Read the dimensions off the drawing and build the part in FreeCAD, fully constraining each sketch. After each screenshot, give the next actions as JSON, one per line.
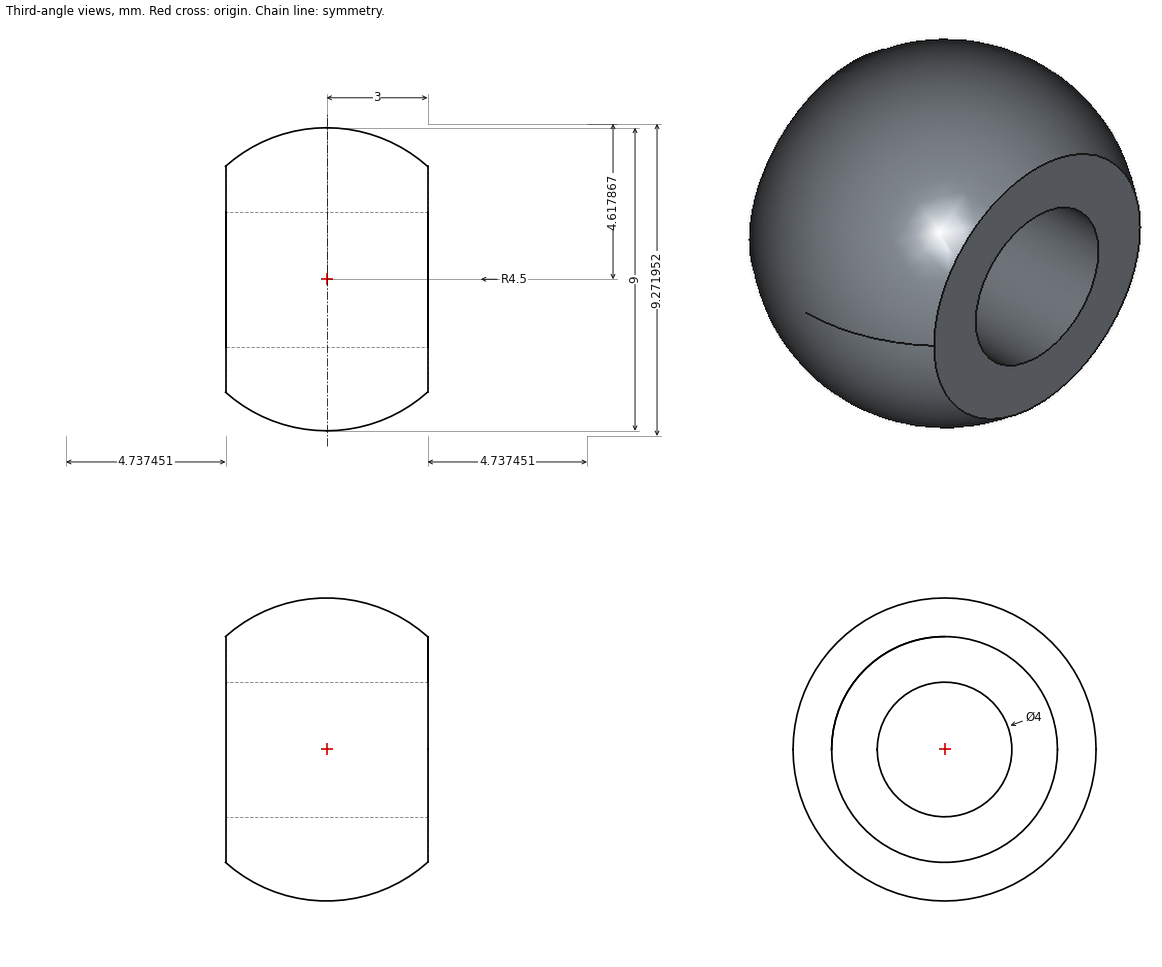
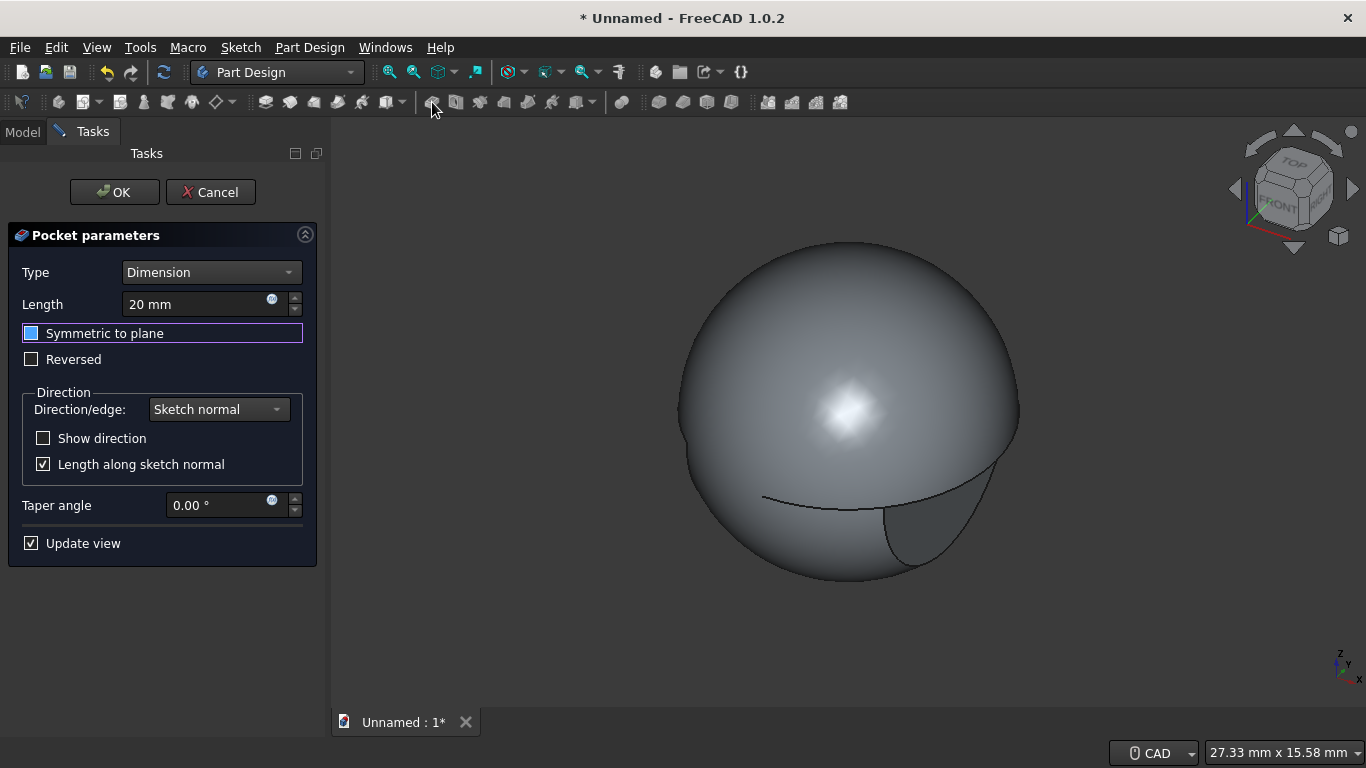
{"action": "left_click", "coordinate": [30, 333]}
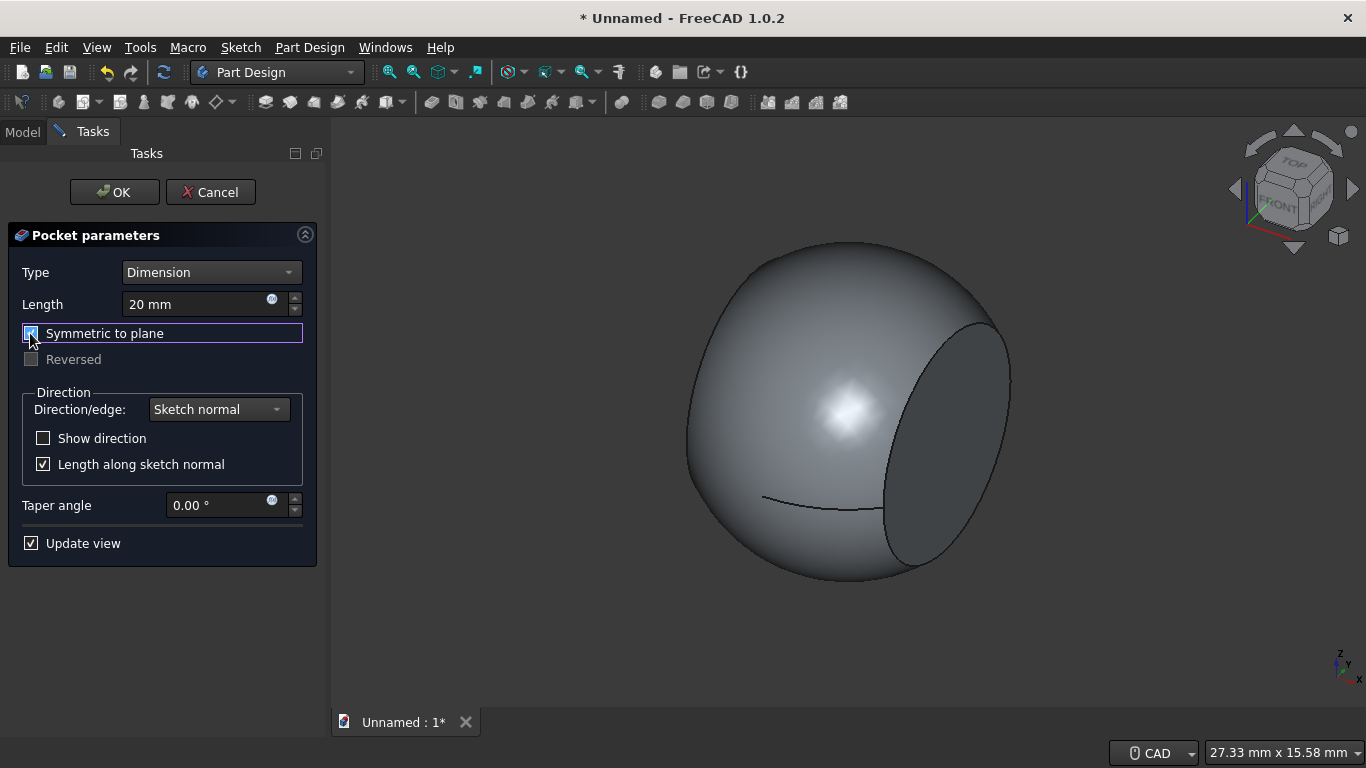
{"action": "left_click", "coordinate": [115, 192]}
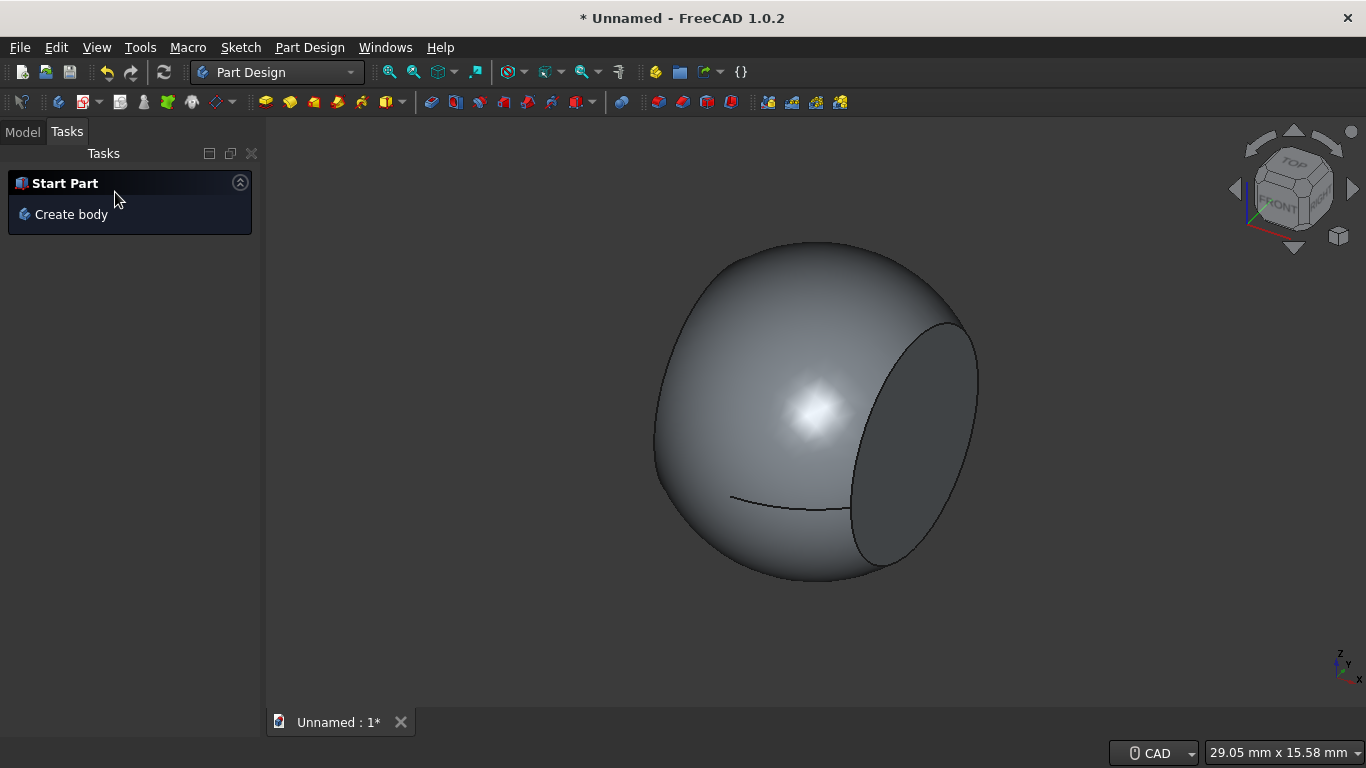
{"action": "key", "text": "6"}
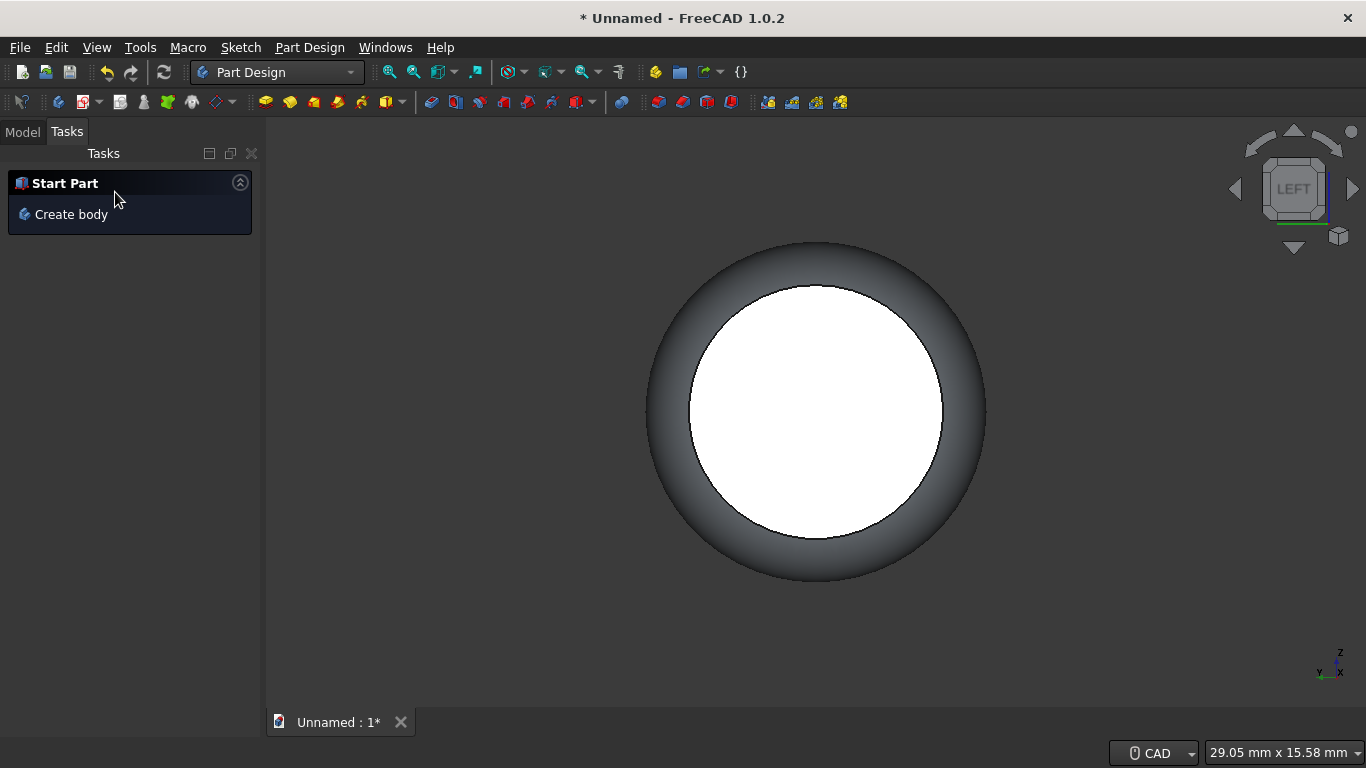
{"action": "left_click", "coordinate": [816, 411]}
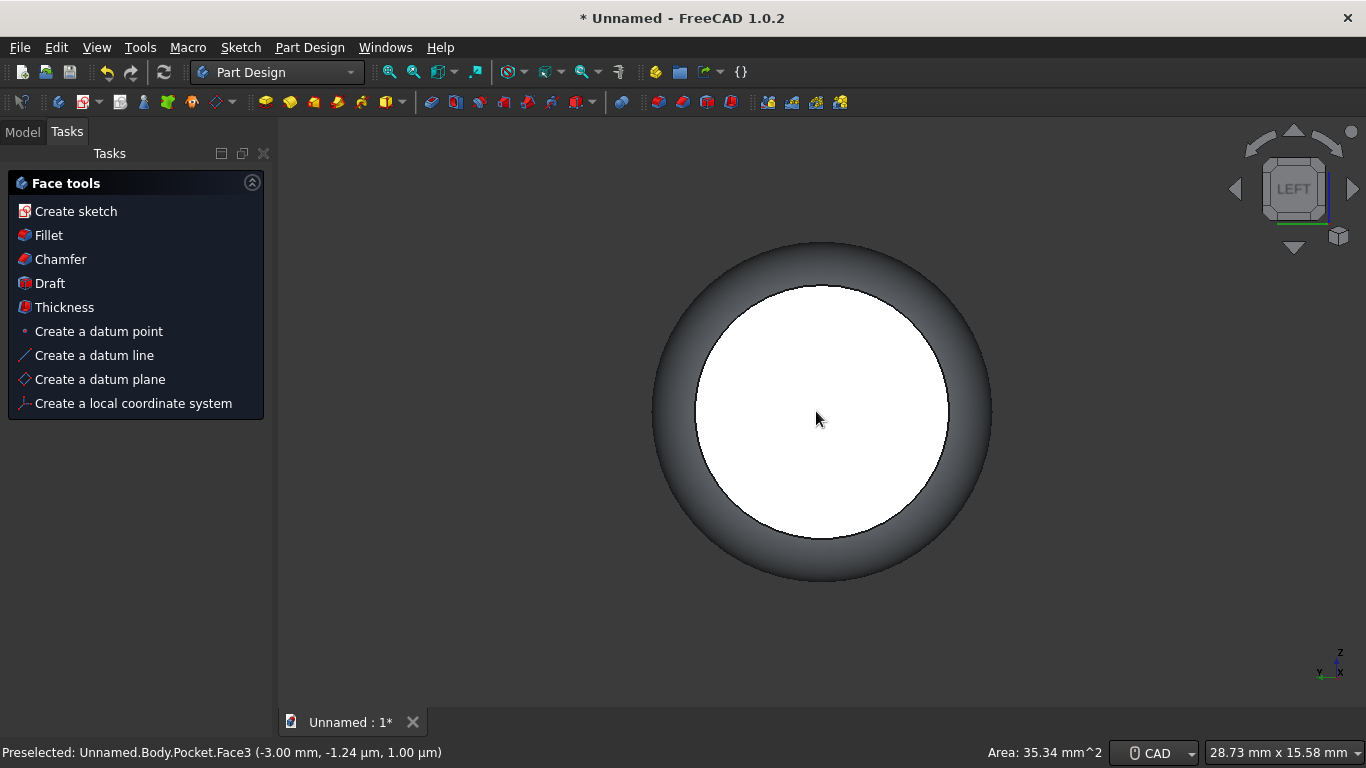
{"action": "left_click", "coordinate": [84, 102]}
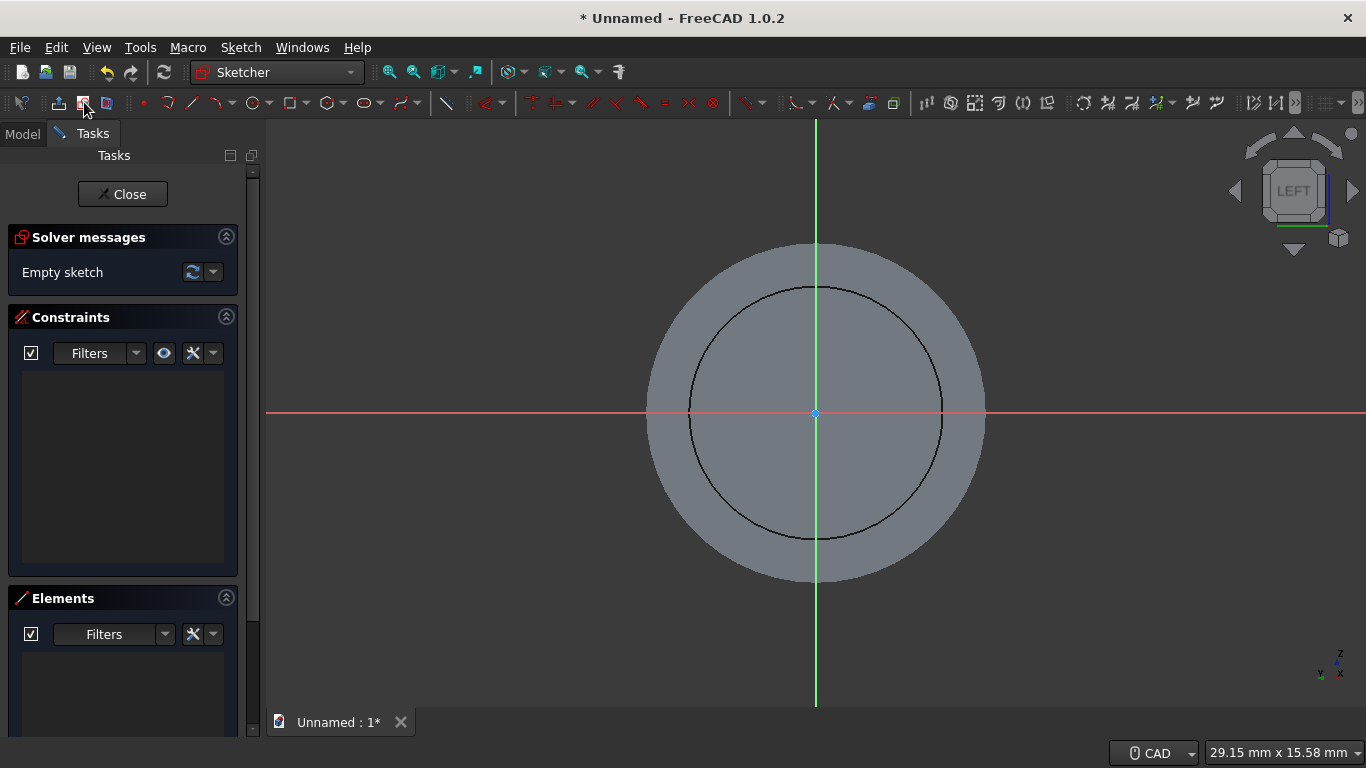
{"action": "scroll", "coordinate": [856, 413], "scroll_direction": "up", "scroll_amount": 5}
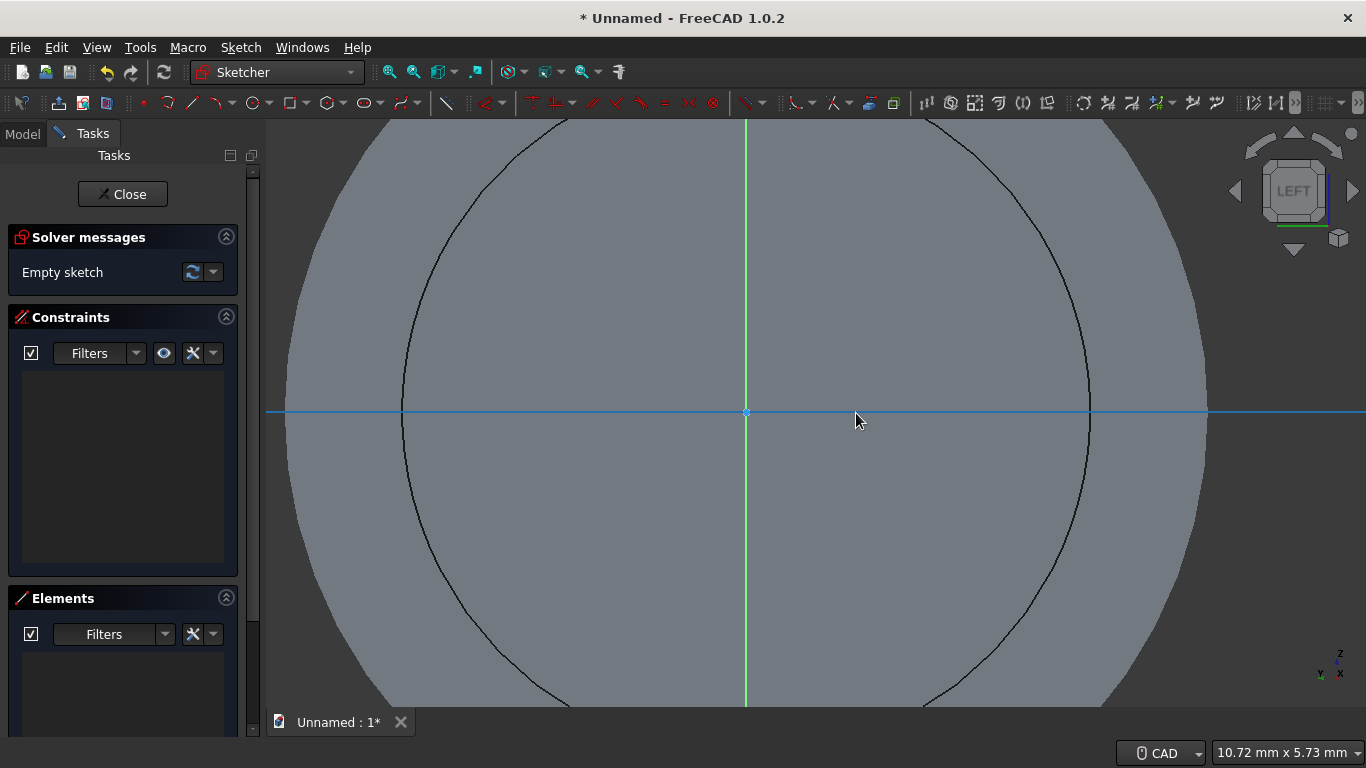
{"action": "key", "text": "g c"}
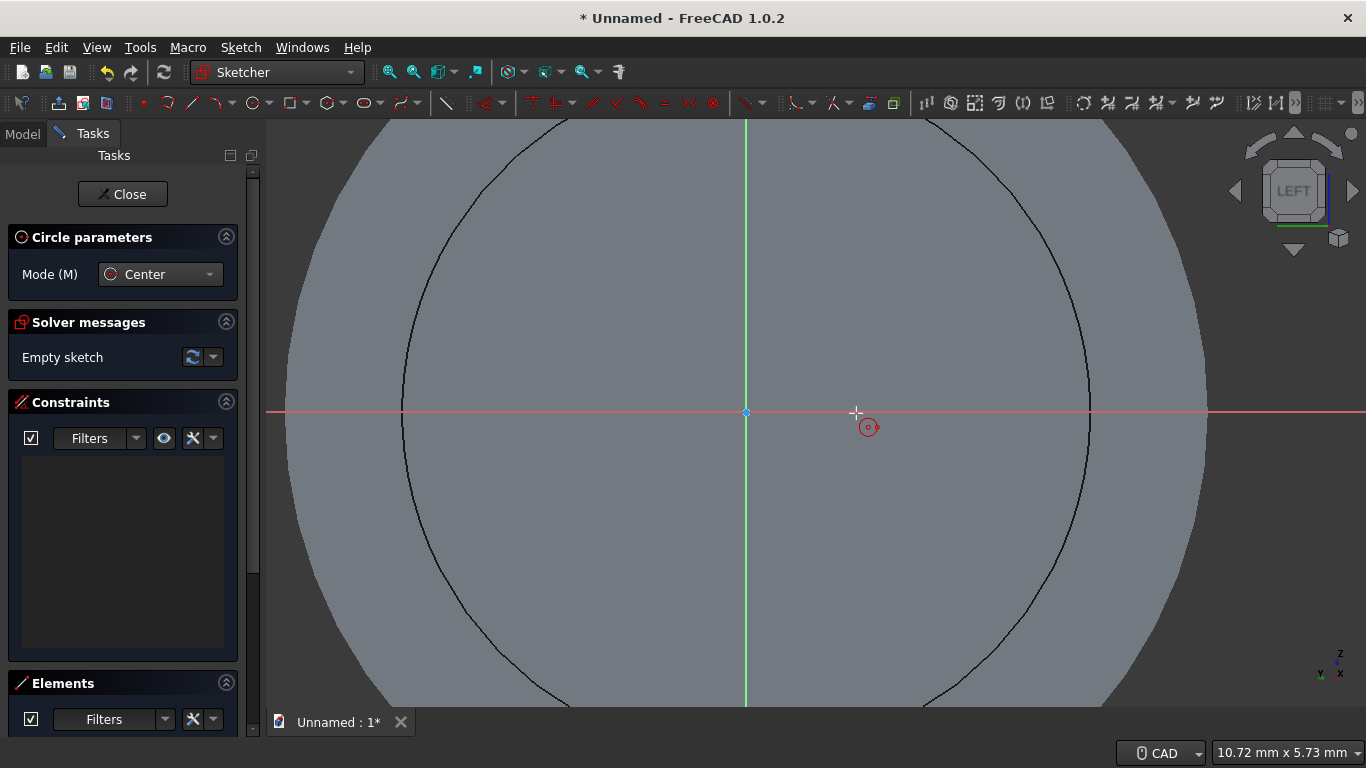
{"action": "left_click", "coordinate": [746, 412]}
{"action": "mouse_move", "coordinate": [891, 267]}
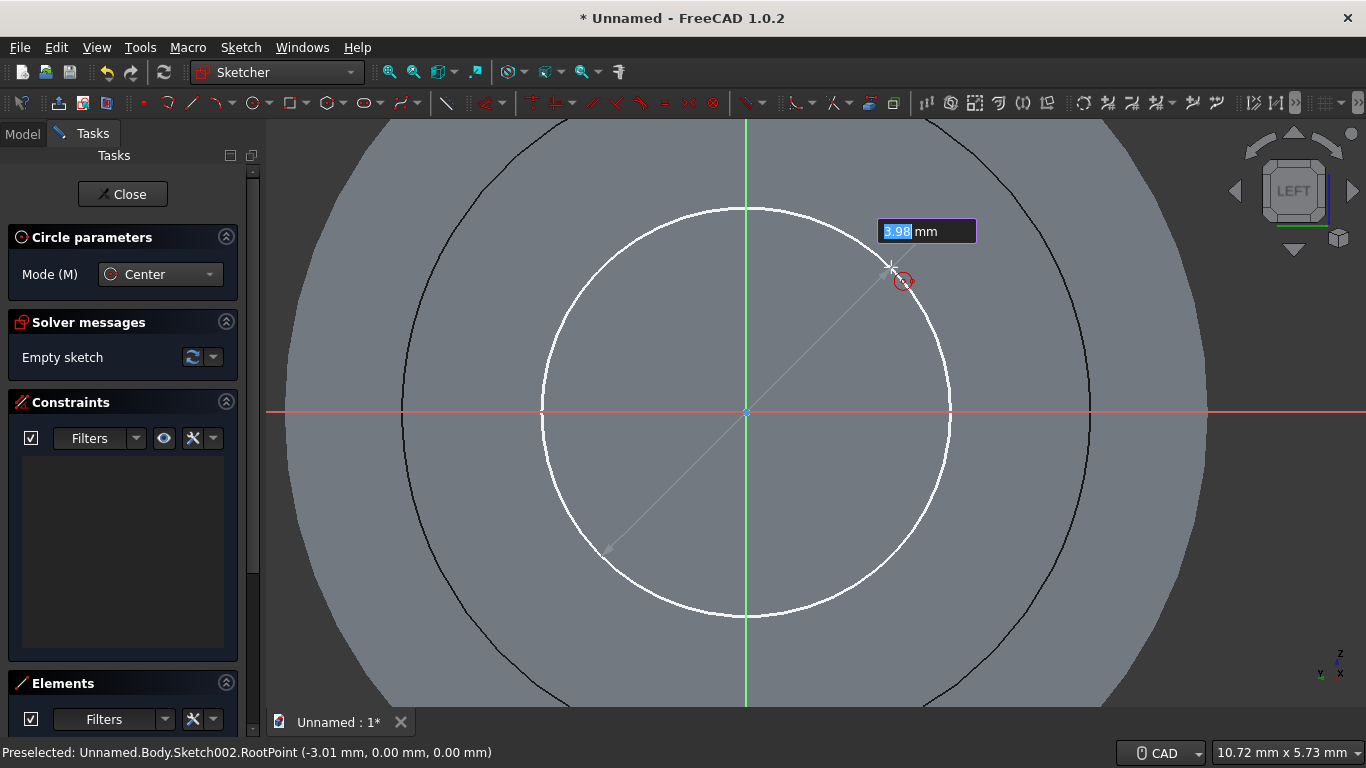
{"action": "type", "text": "4"}
{"action": "key", "text": "Return"}
{"action": "key", "text": "Escape"}